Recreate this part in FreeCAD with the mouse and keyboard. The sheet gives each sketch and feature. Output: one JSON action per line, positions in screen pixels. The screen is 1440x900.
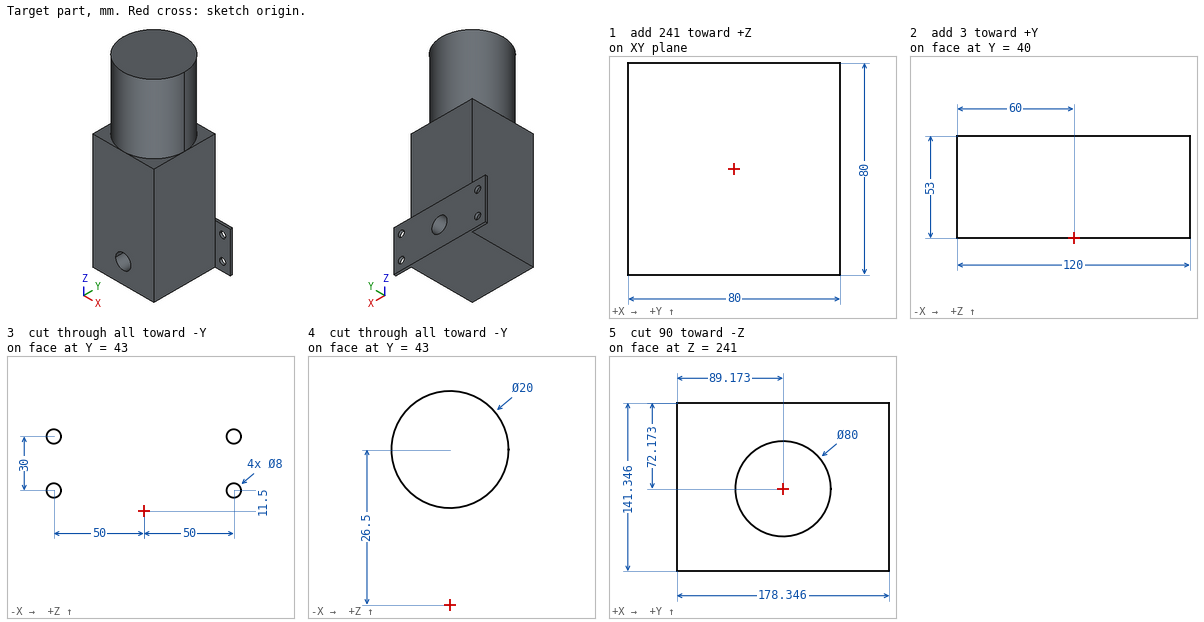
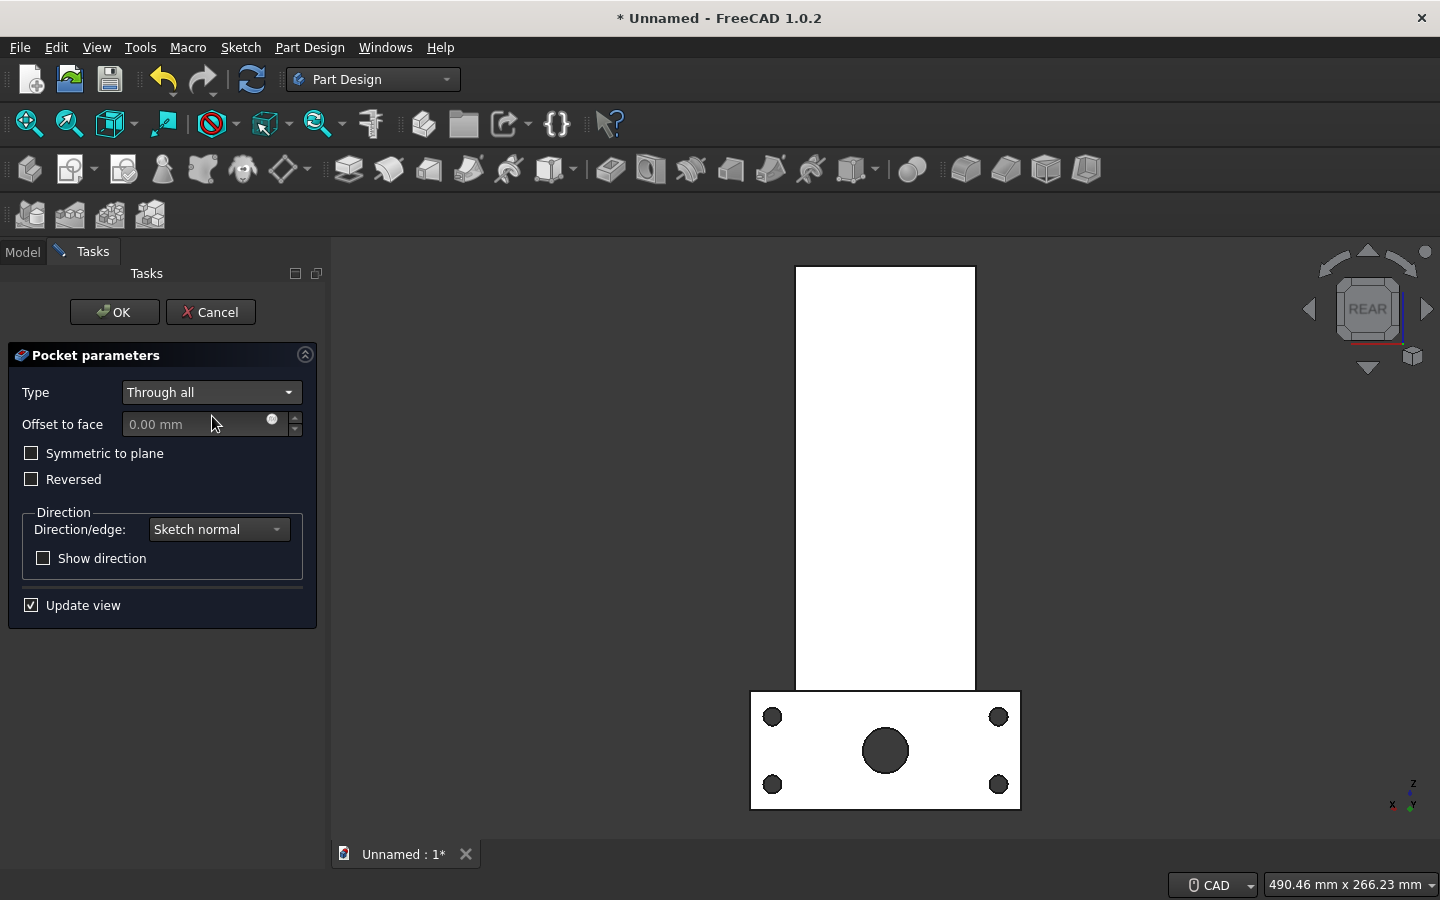
{"action": "left_click", "coordinate": [115, 312]}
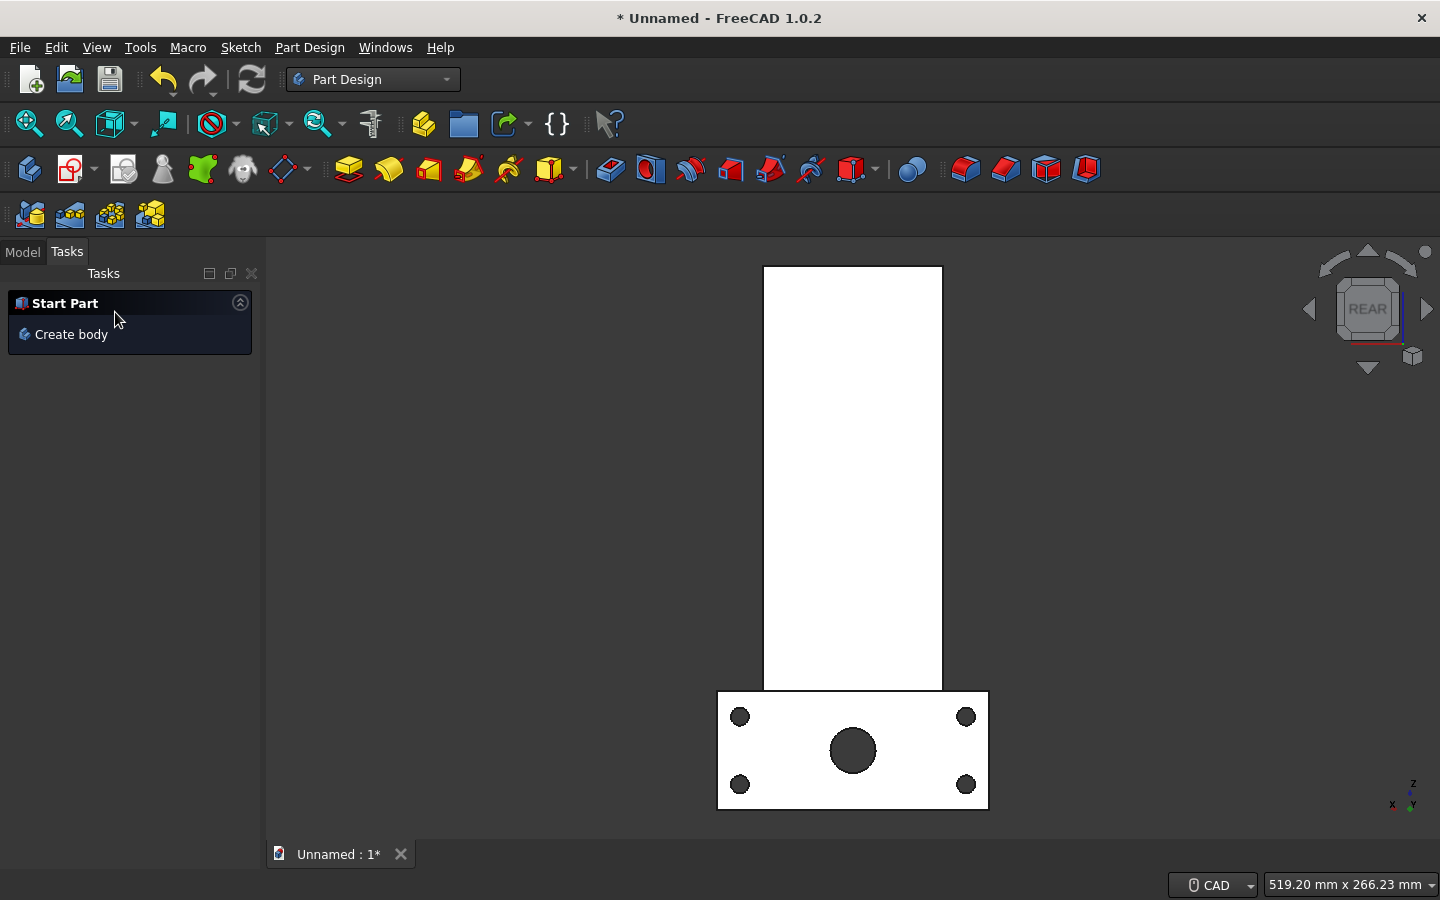
{"action": "key", "text": "0"}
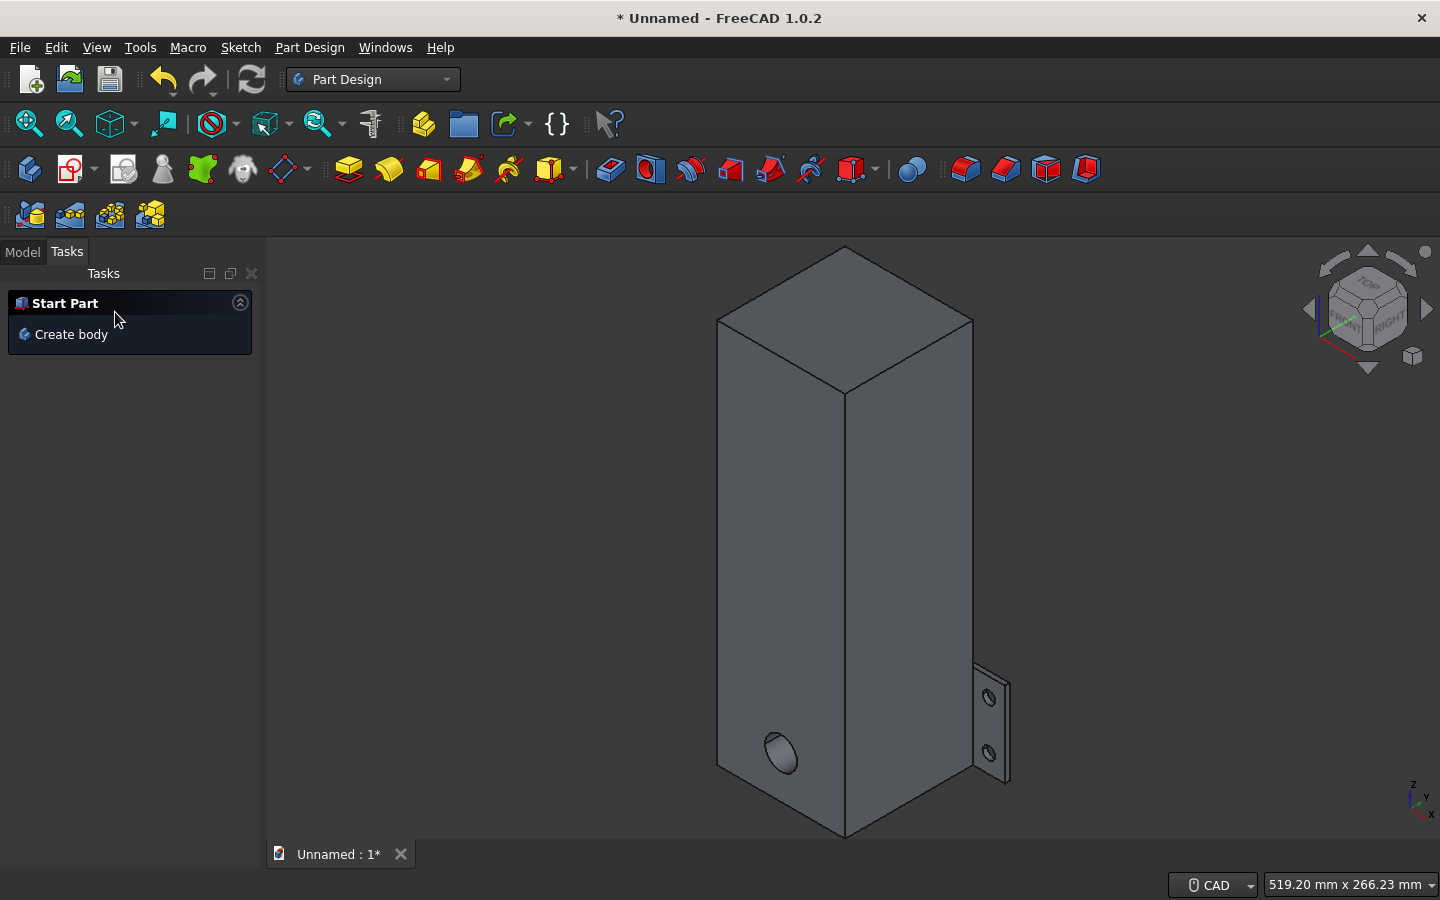
{"action": "key", "text": "v f"}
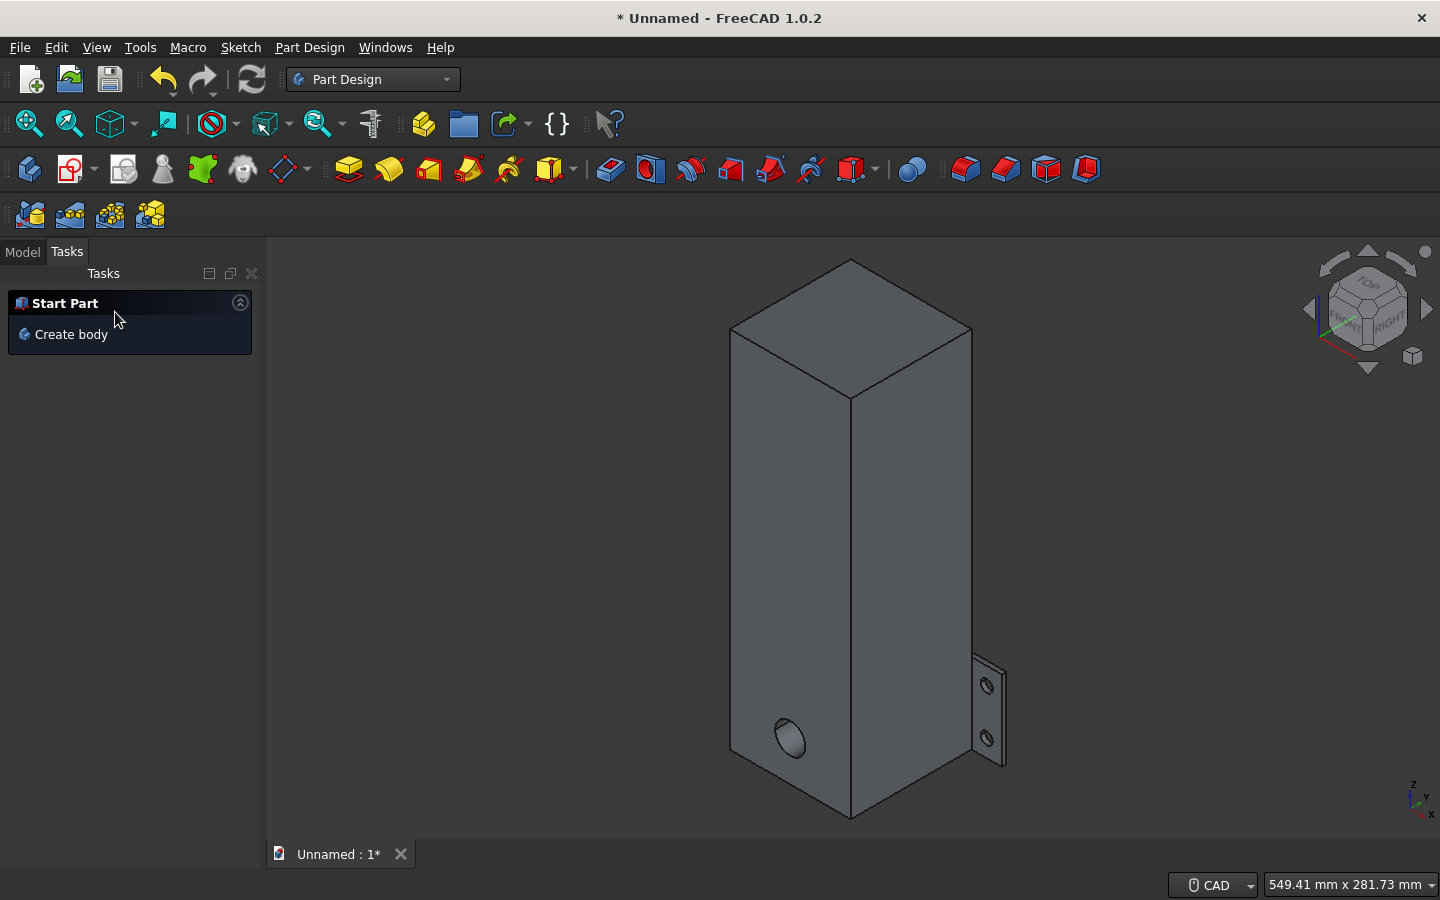
{"action": "left_click", "coordinate": [851, 328]}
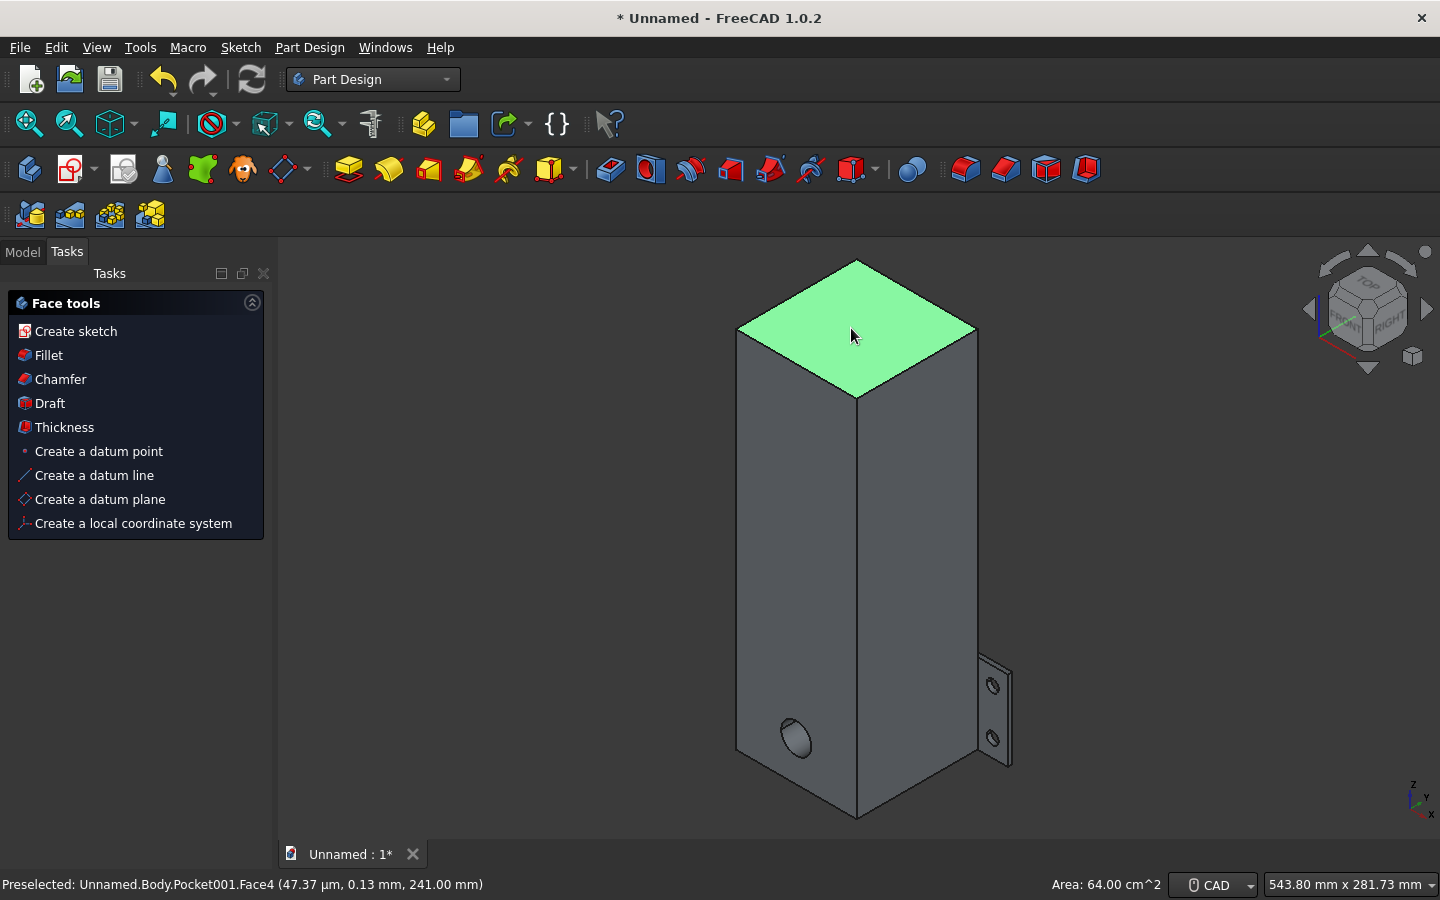
{"action": "left_click", "coordinate": [70, 170]}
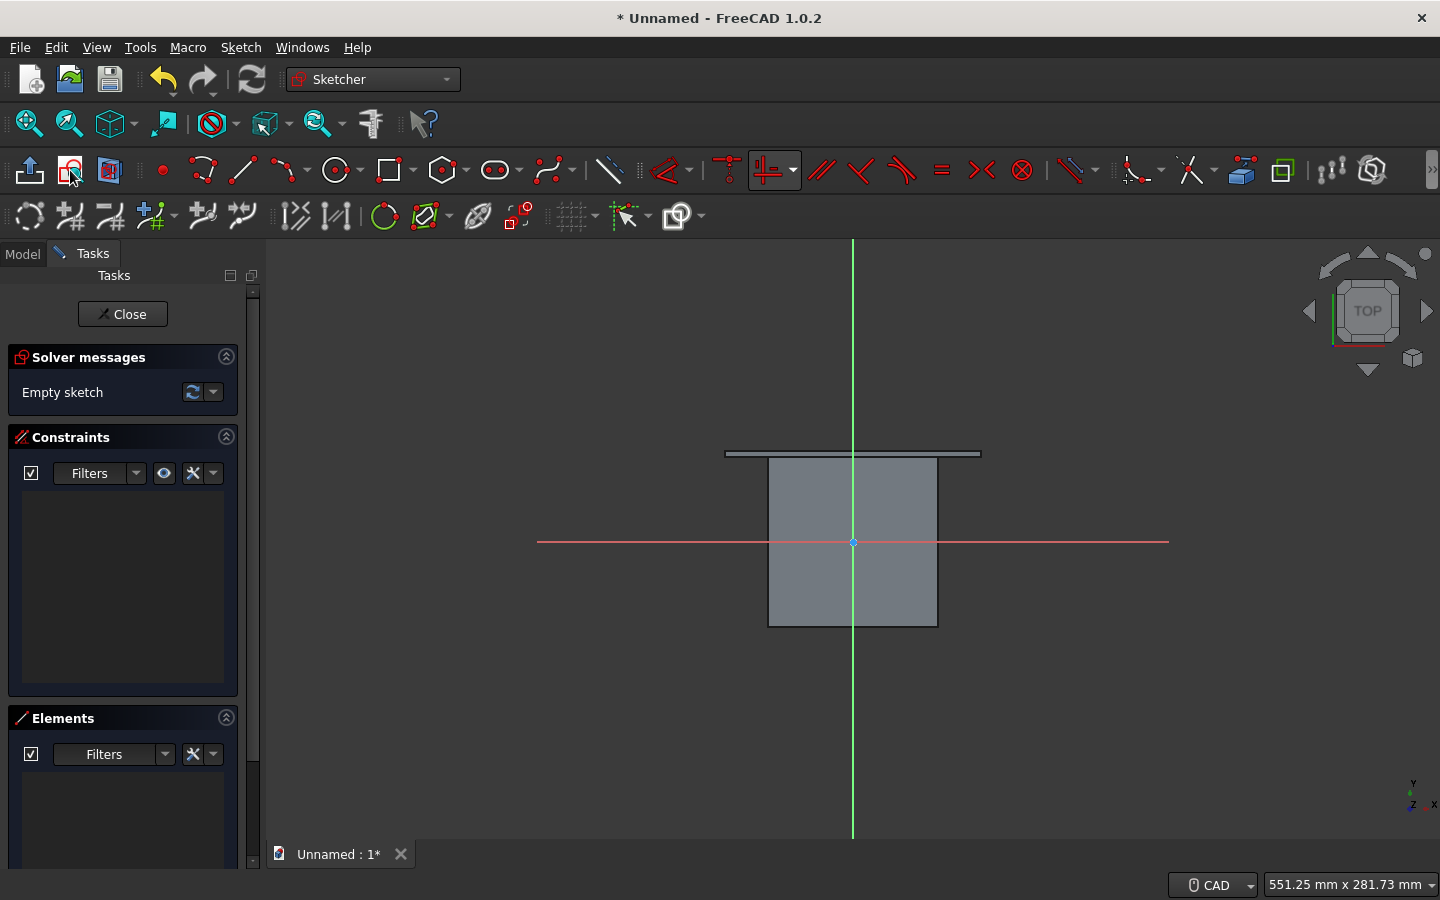
{"action": "left_click", "coordinate": [390, 170]}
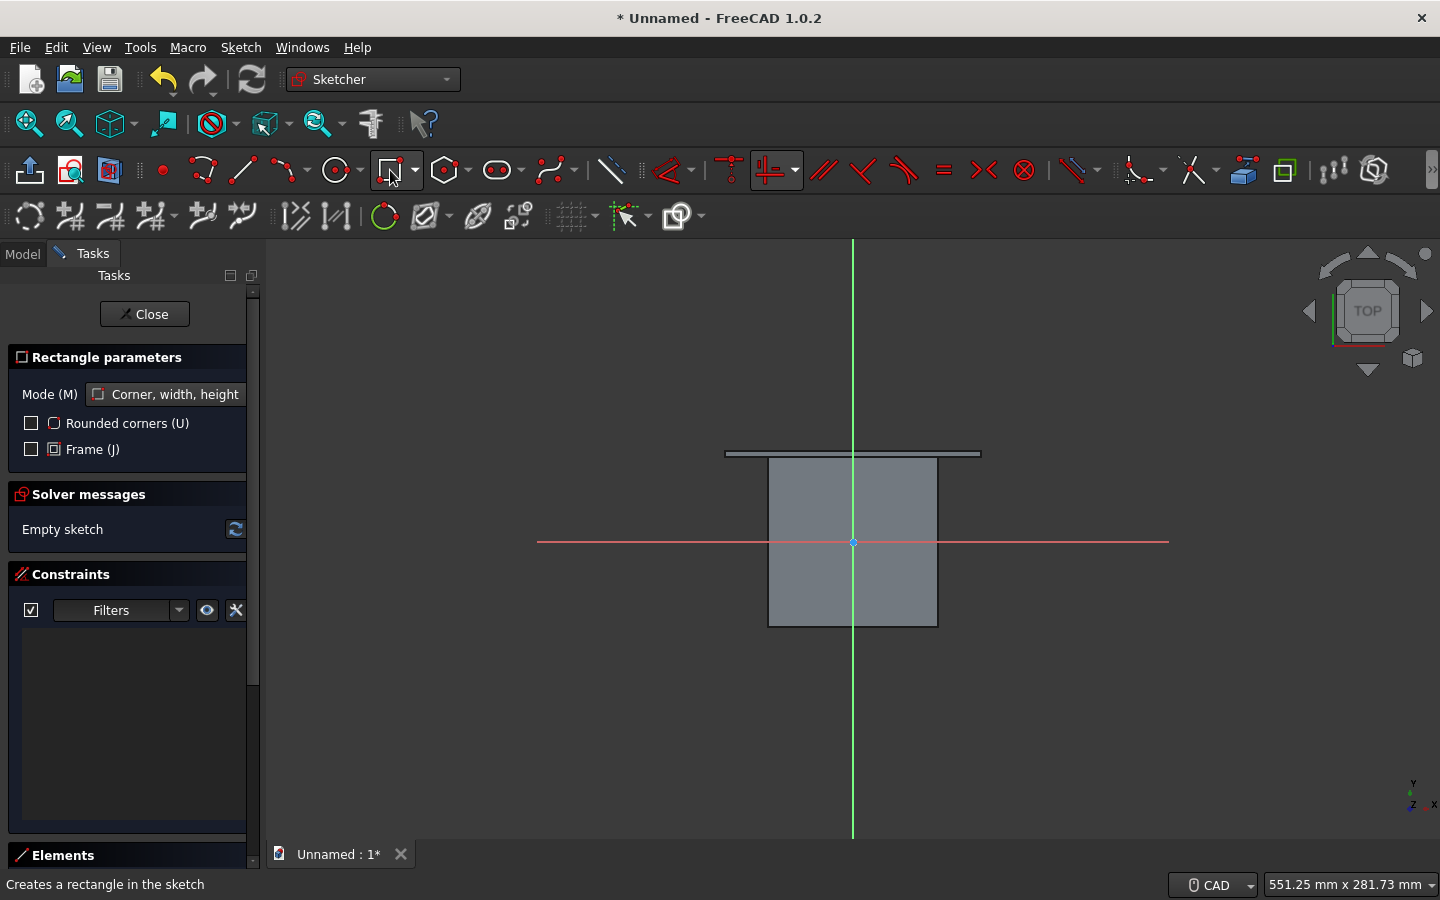
{"action": "left_click", "coordinate": [663, 388]}
{"action": "left_click", "coordinate": [1043, 690]}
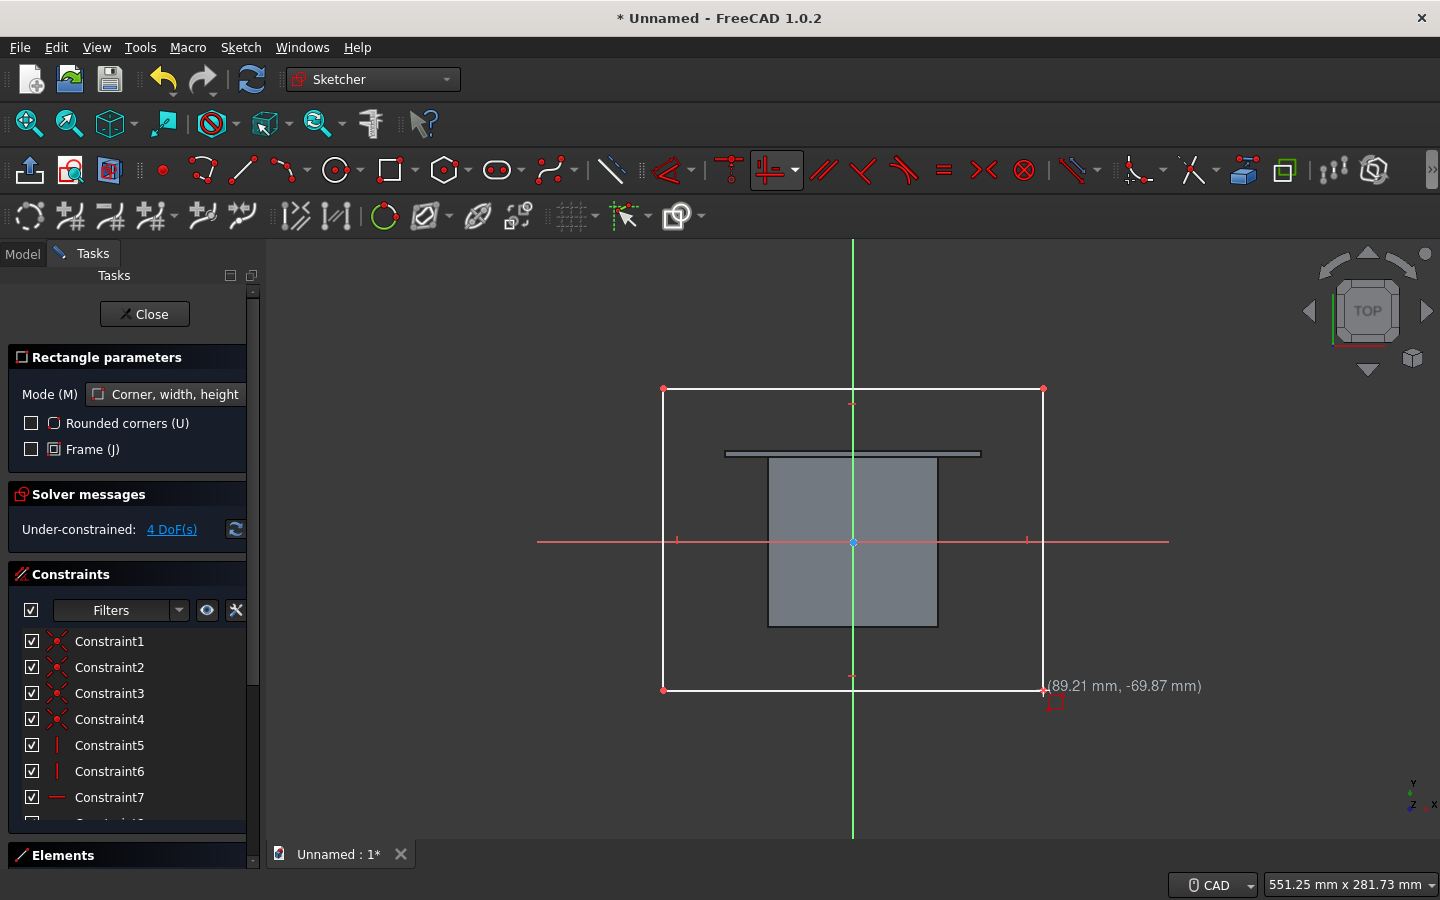
{"action": "left_click", "coordinate": [336, 170]}